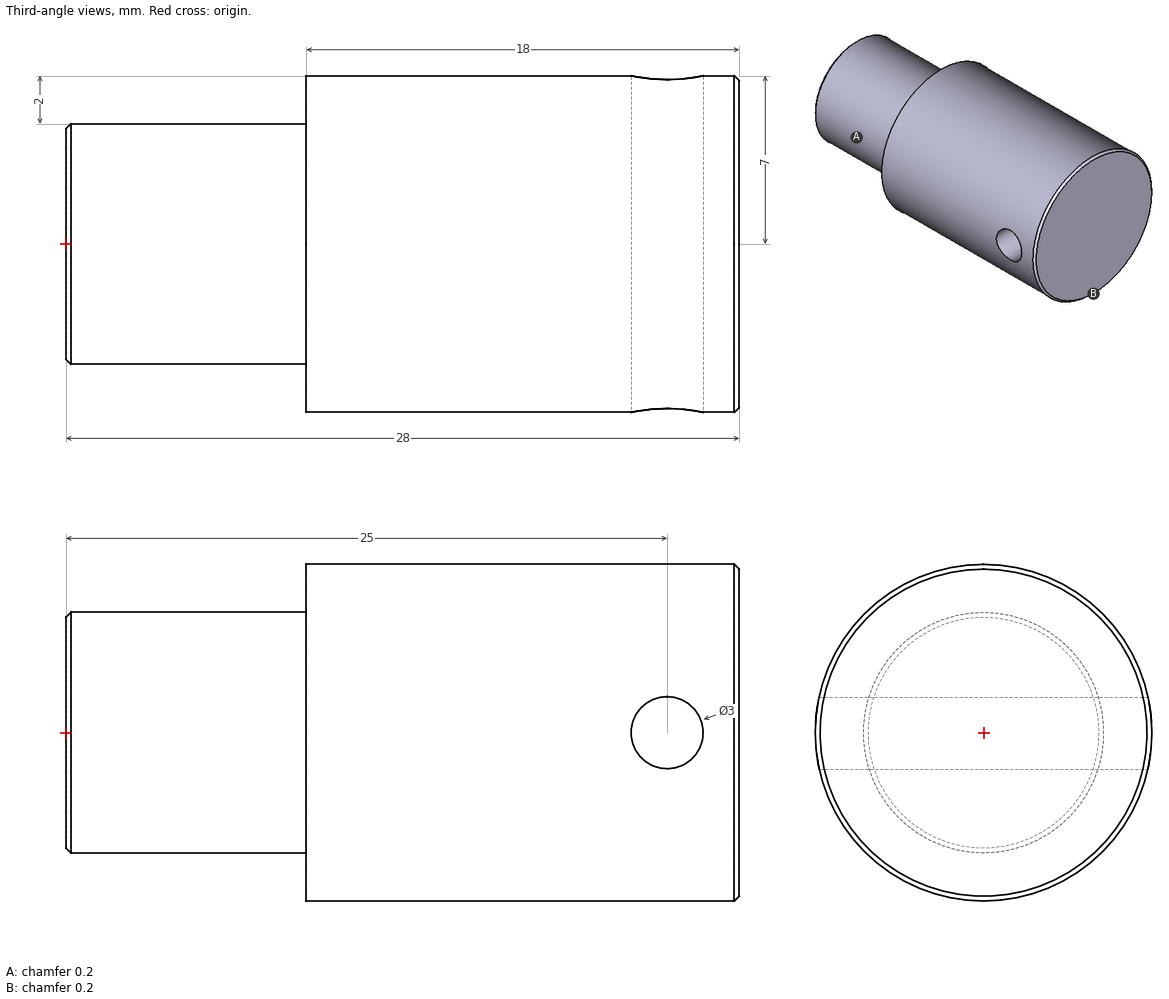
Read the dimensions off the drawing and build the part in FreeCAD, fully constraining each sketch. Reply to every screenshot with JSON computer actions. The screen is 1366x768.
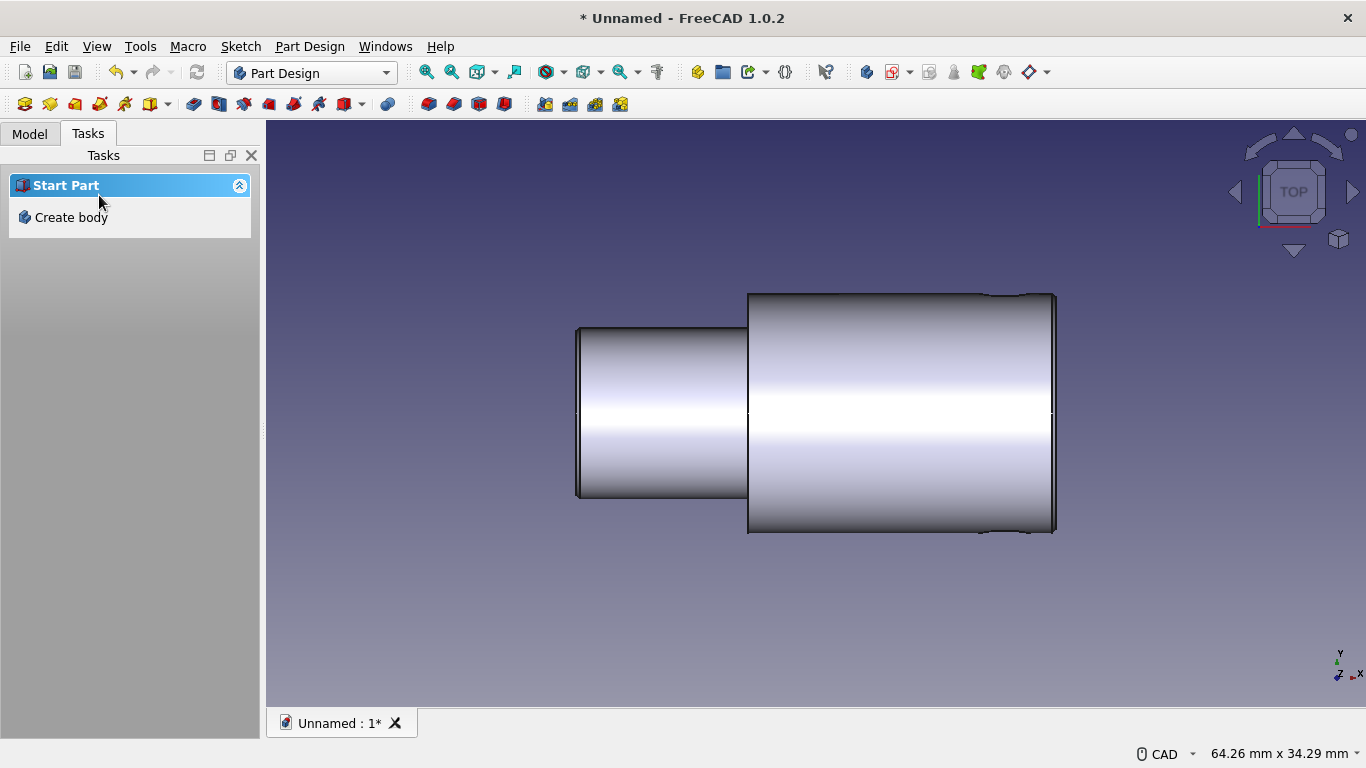
{"action": "key", "text": "0"}